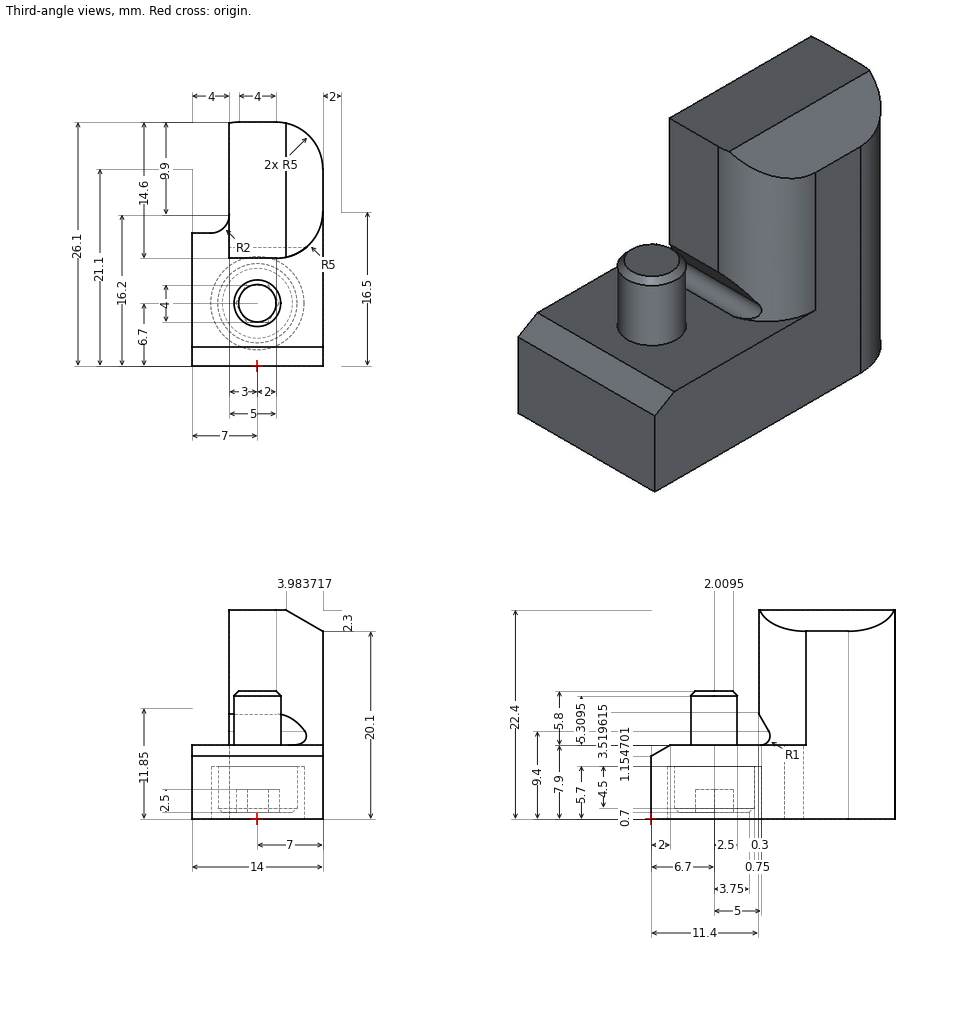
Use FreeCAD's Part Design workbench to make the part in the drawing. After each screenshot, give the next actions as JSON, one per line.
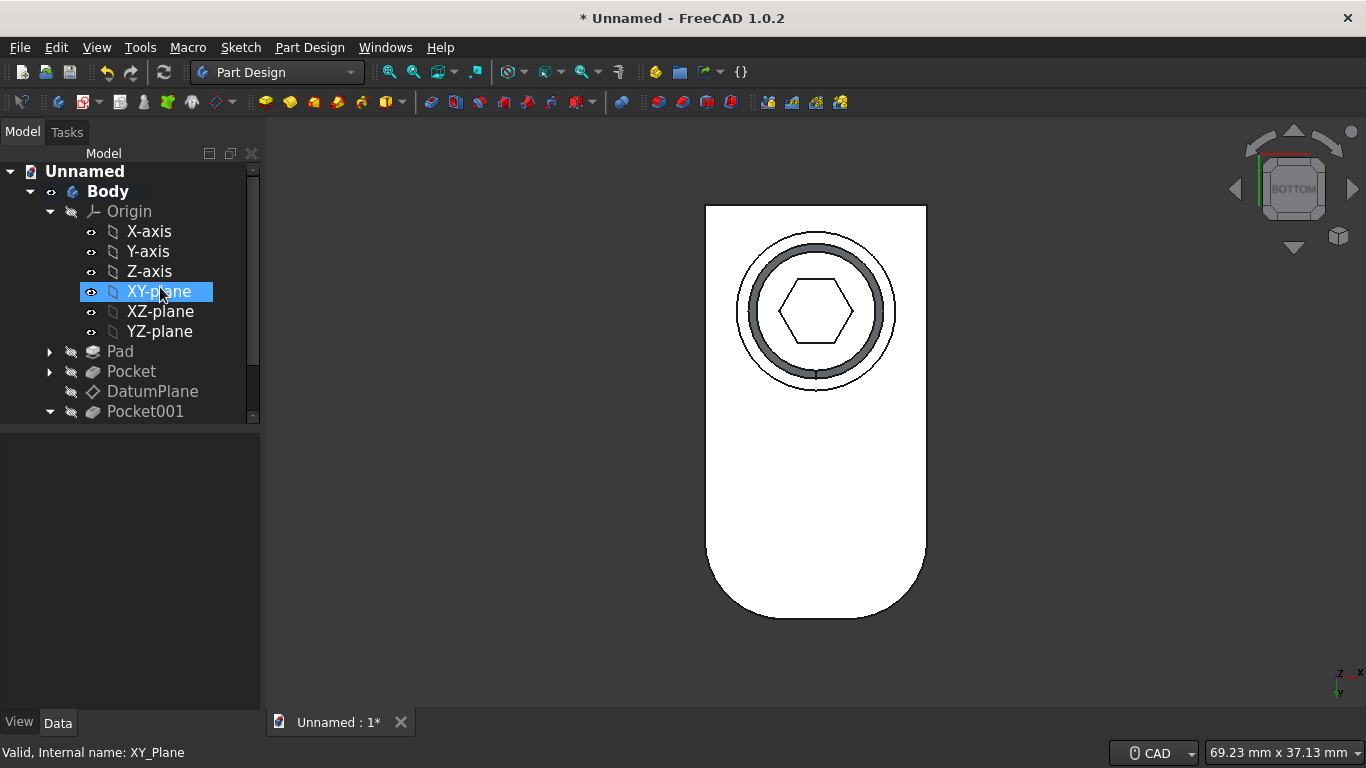
{"action": "left_click", "coordinate": [136, 292]}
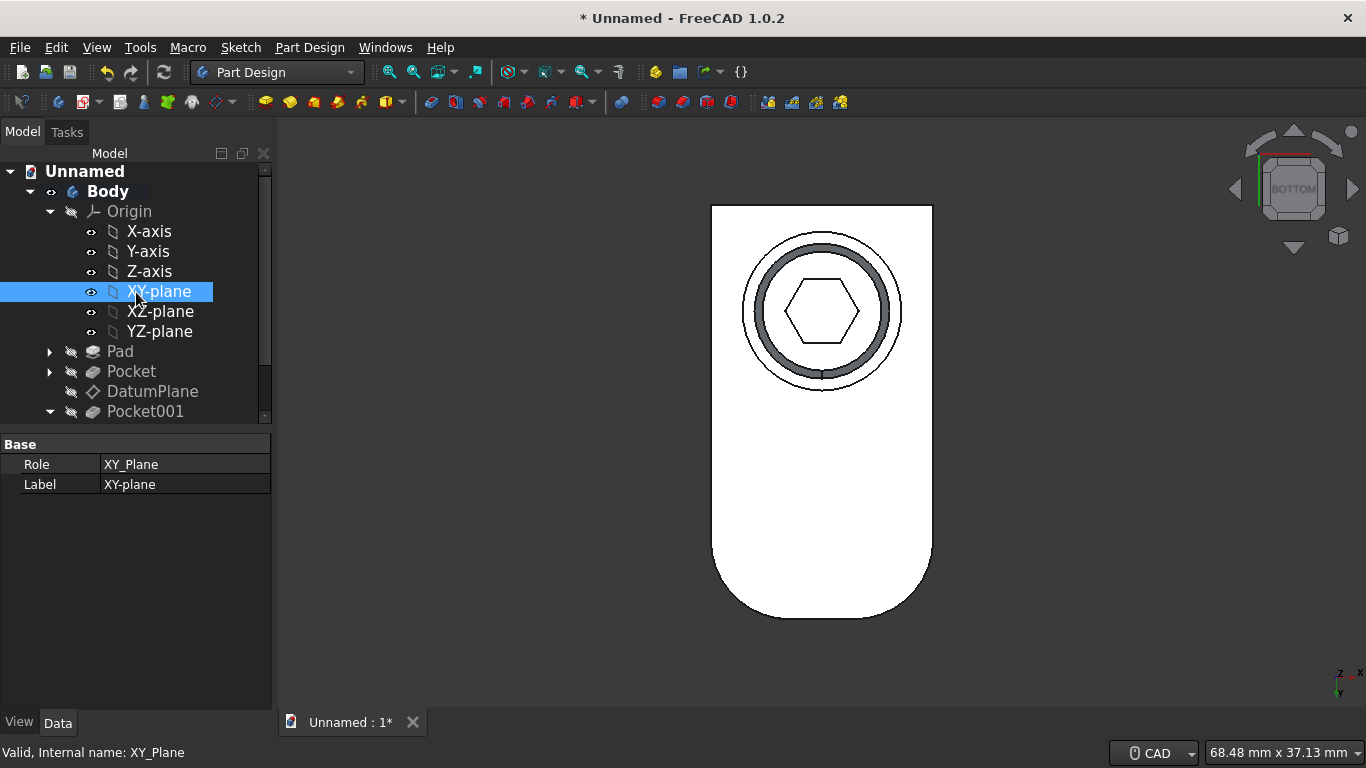
{"action": "left_click", "coordinate": [216, 102]}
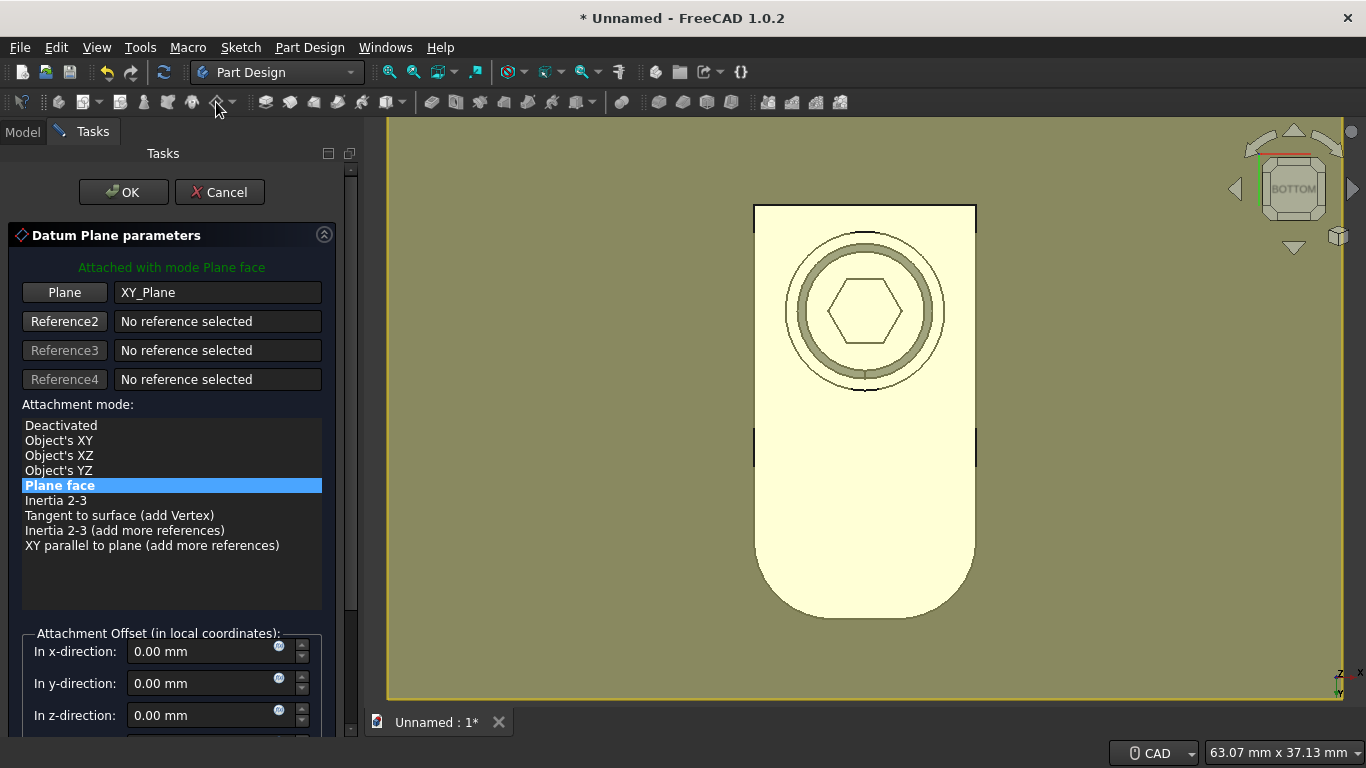
{"action": "triple_click", "coordinate": [210, 715]}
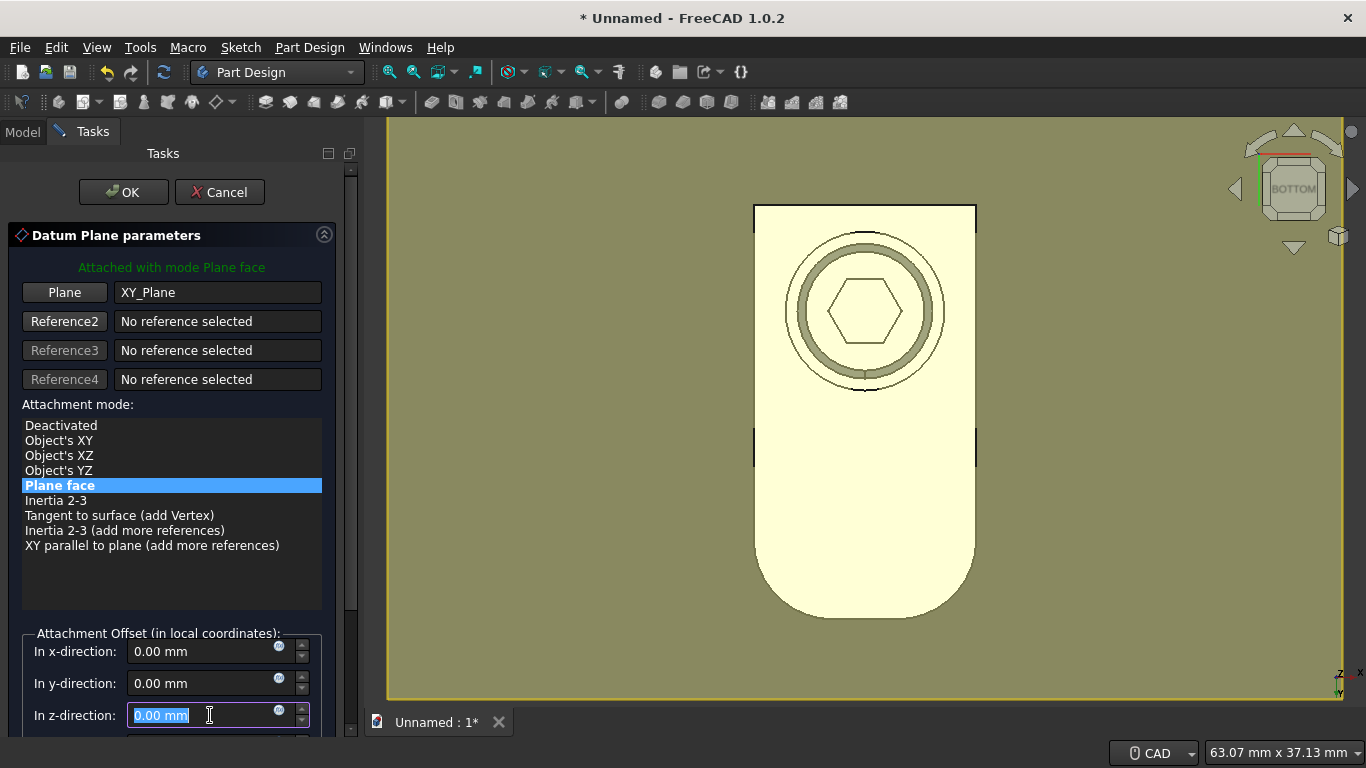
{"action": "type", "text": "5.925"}
{"action": "key", "text": "Tab"}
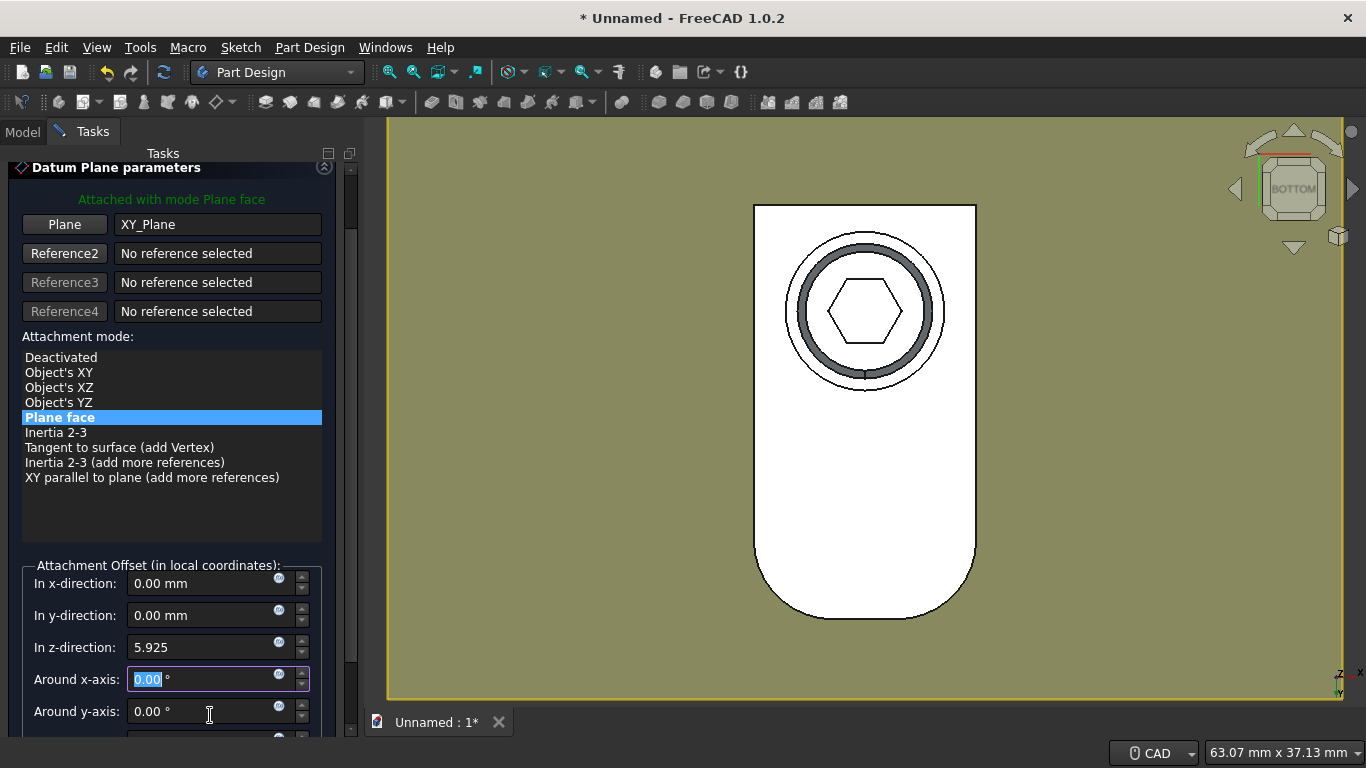
{"action": "scroll", "coordinate": [351, 450], "scroll_direction": "up", "scroll_amount": 2}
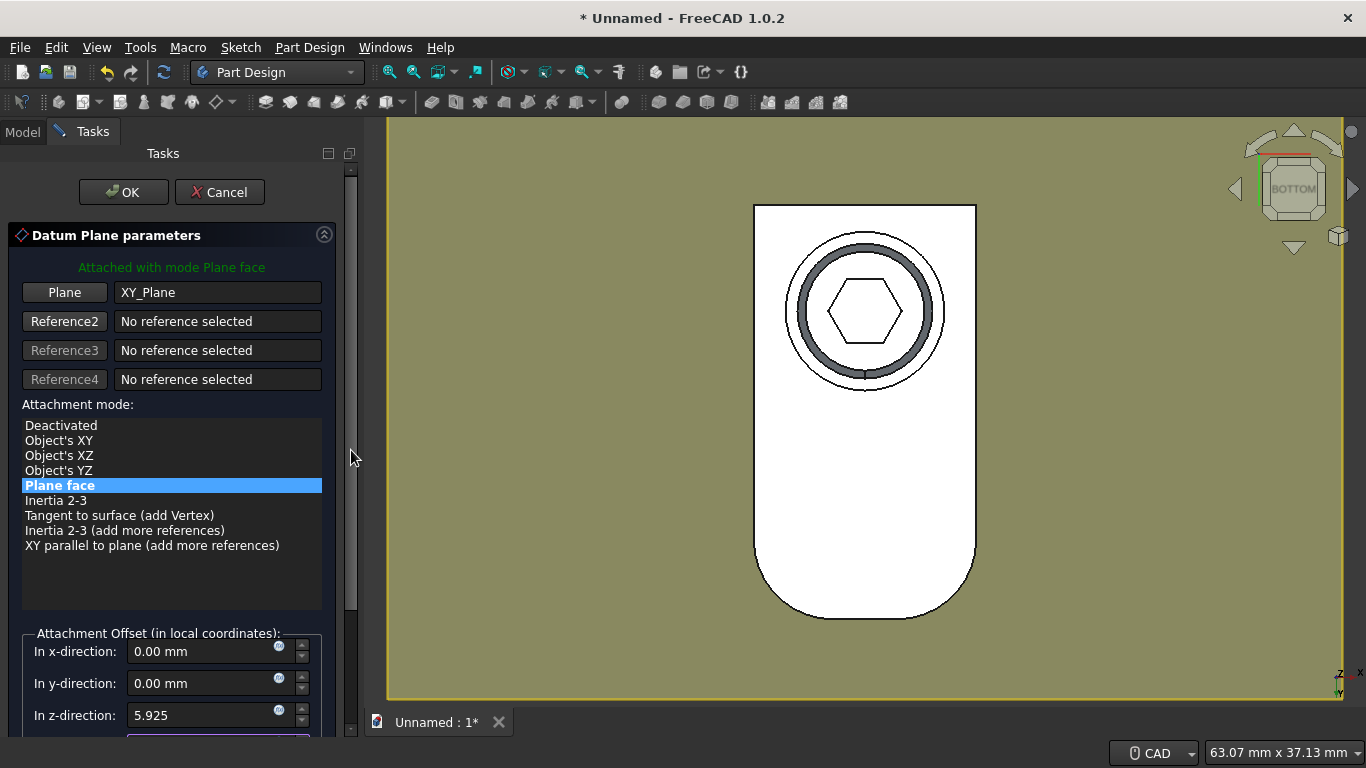
{"action": "left_click", "coordinate": [124, 192]}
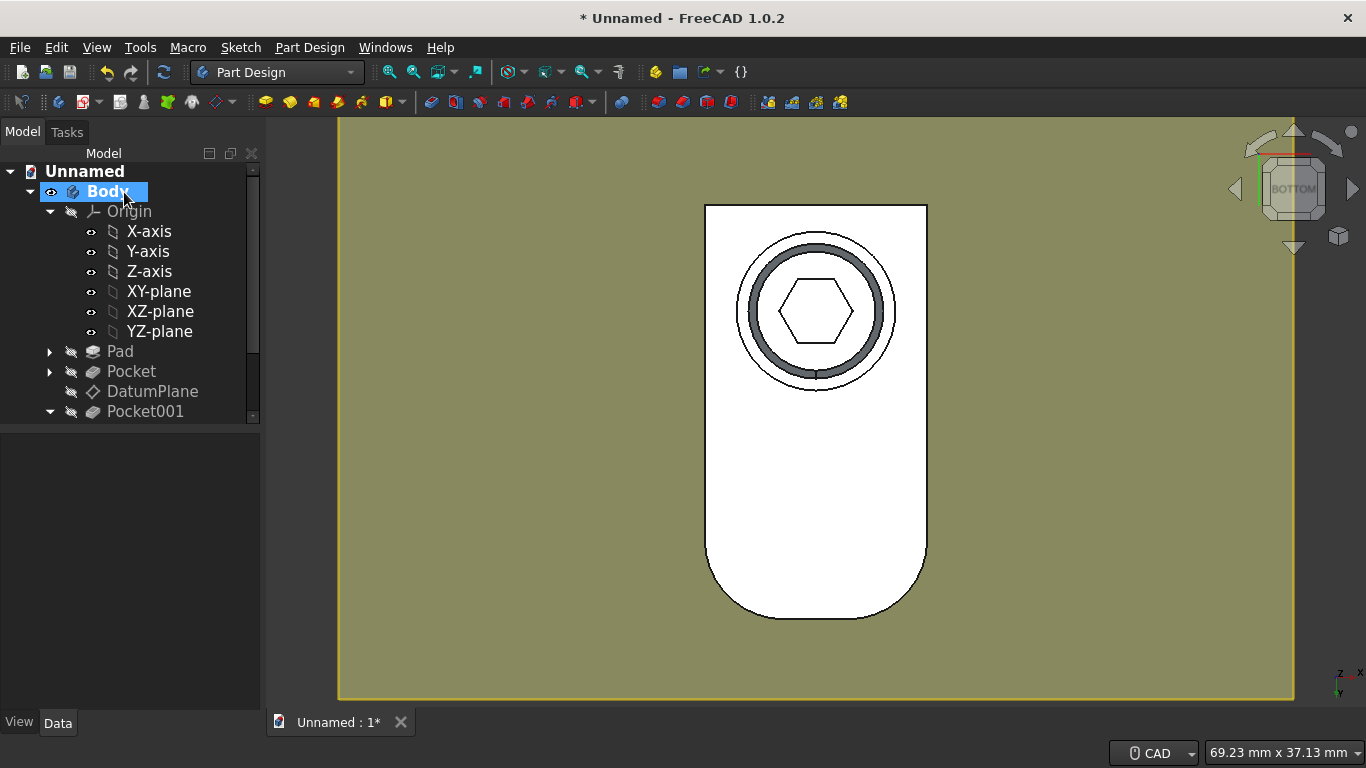
{"action": "scroll", "coordinate": [100, 287], "scroll_direction": "down", "scroll_amount": 3}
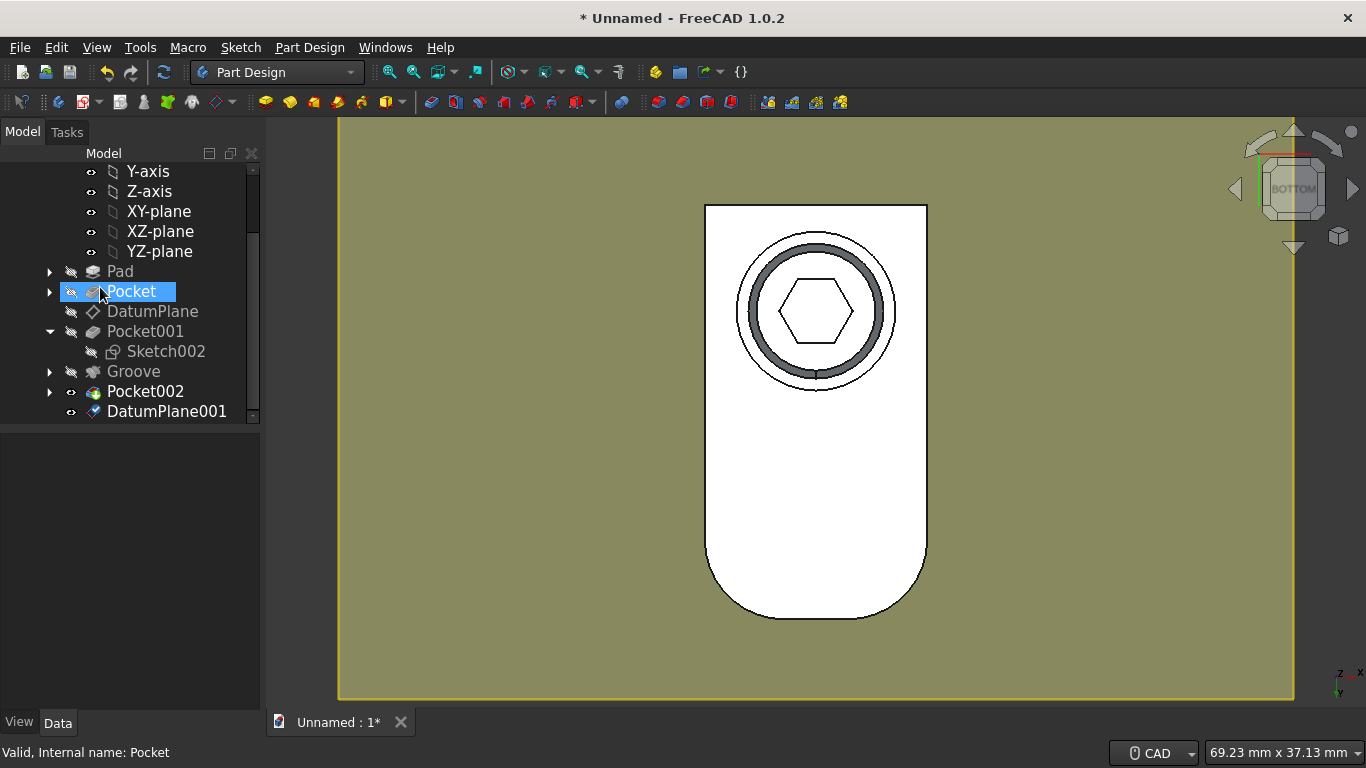
{"action": "left_click", "coordinate": [116, 412]}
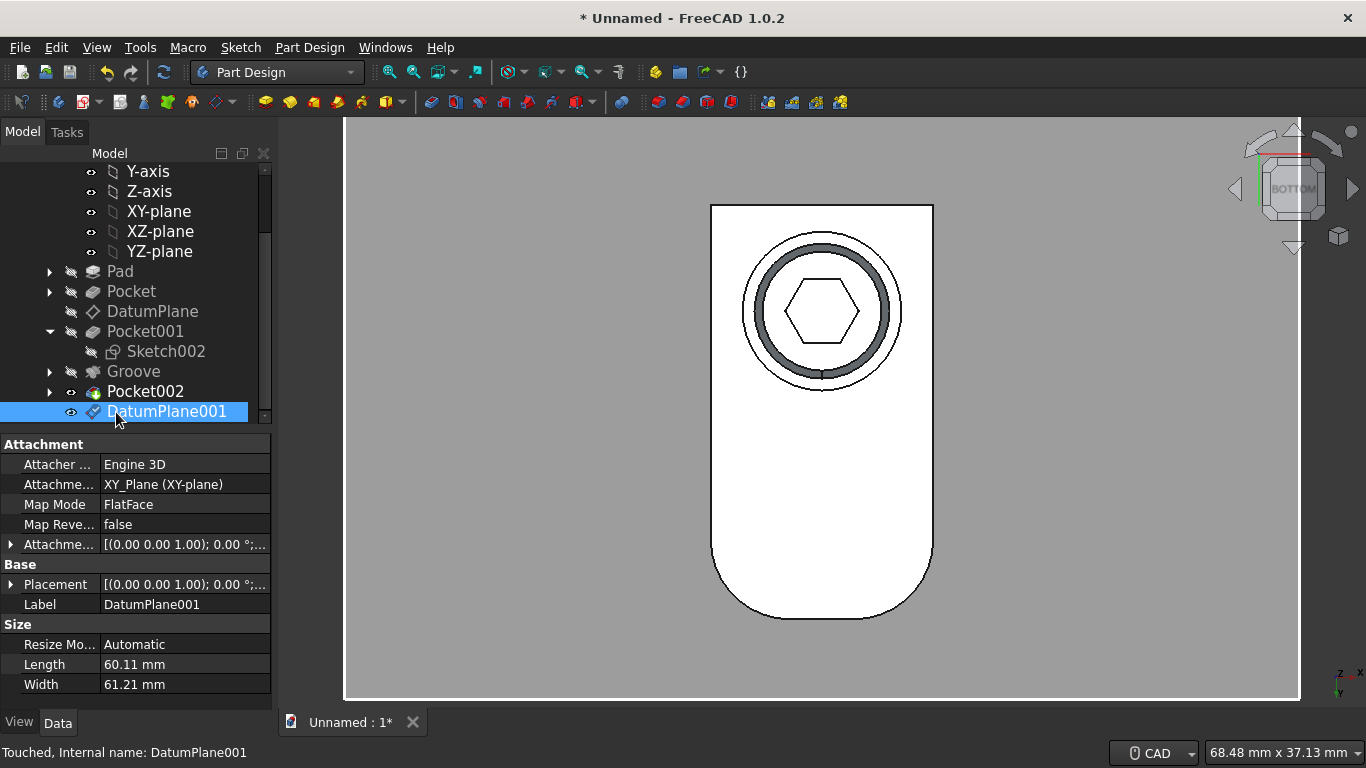
{"action": "left_click", "coordinate": [84, 102]}